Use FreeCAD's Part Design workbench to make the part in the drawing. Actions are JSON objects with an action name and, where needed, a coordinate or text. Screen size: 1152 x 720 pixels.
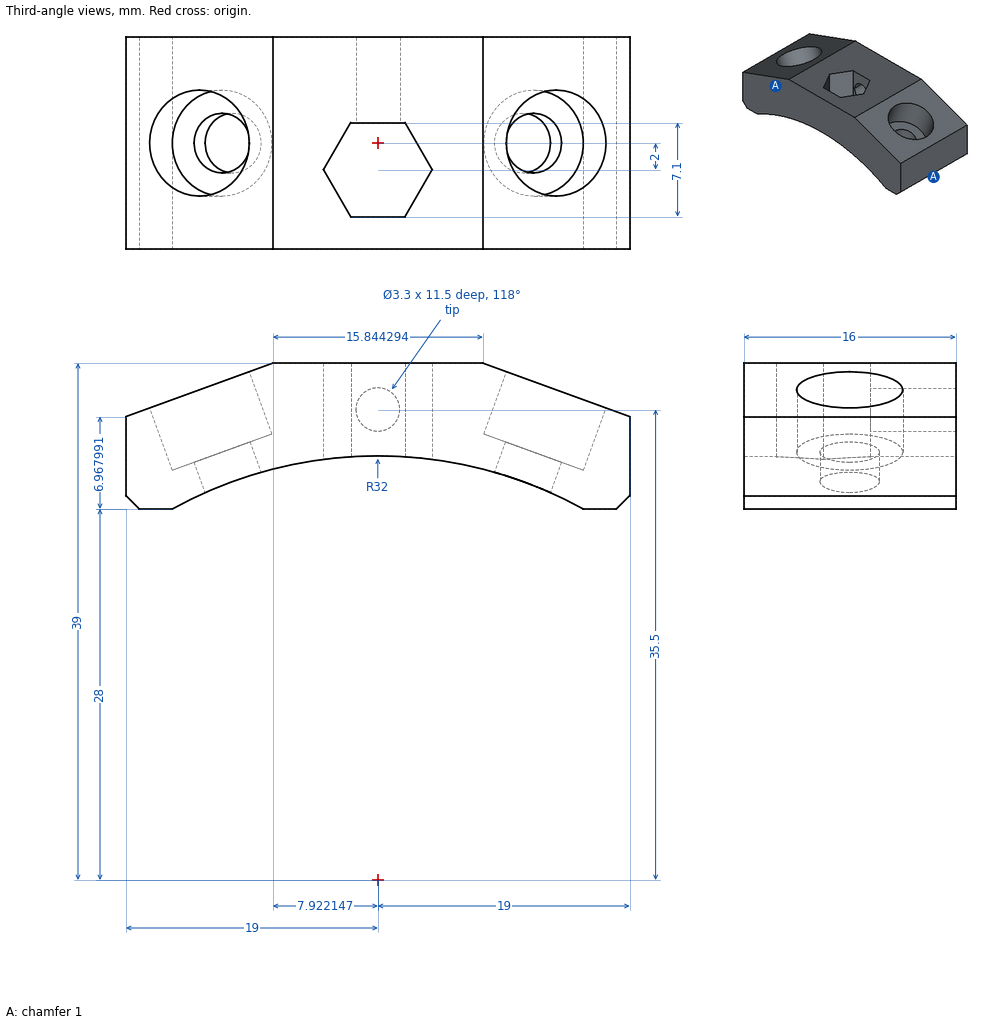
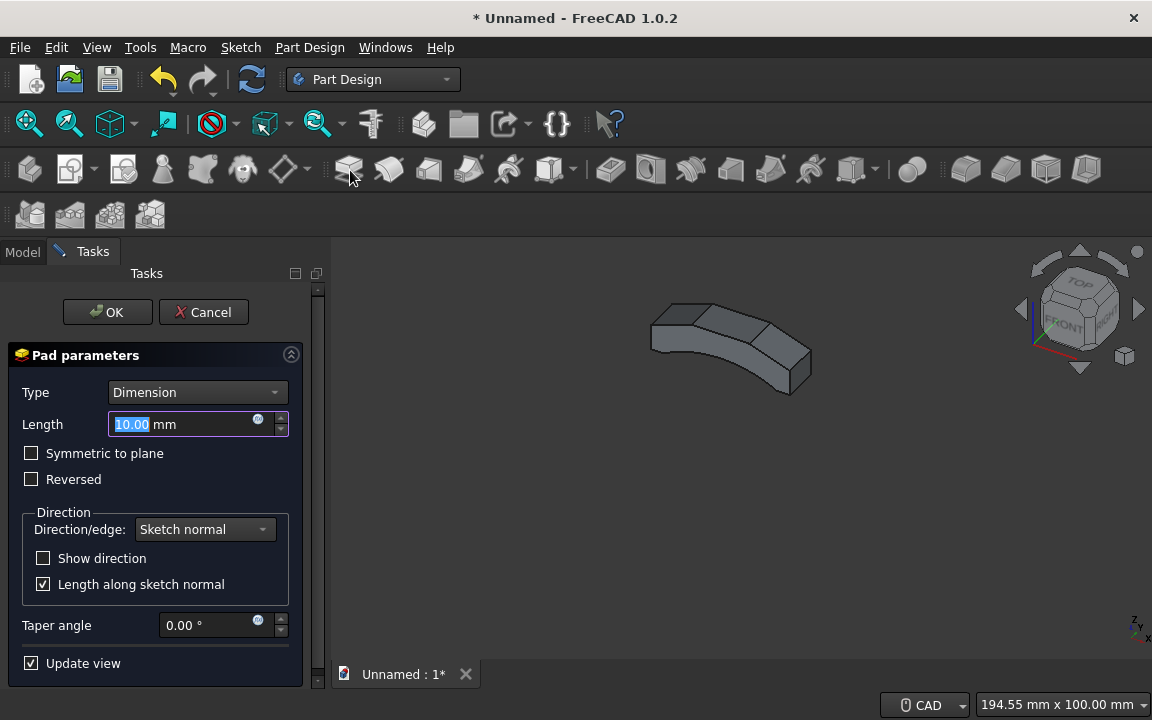
{"action": "type", "text": "16"}
{"action": "key", "text": "Tab"}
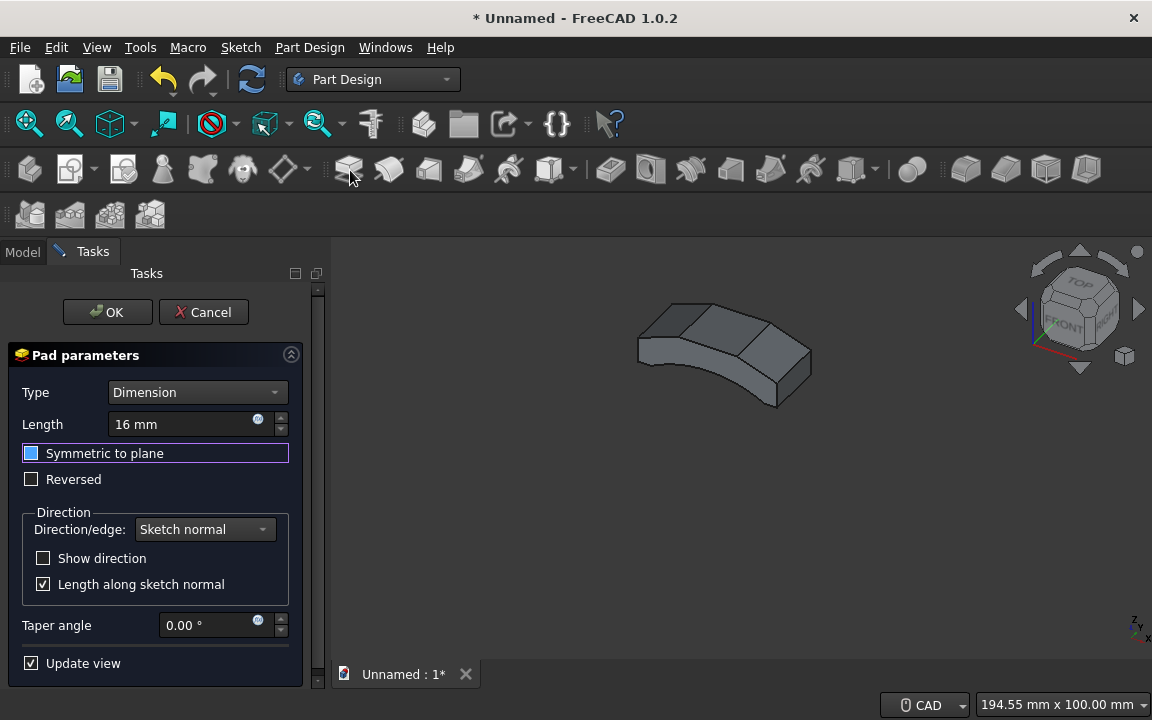
{"action": "left_click", "coordinate": [30, 453]}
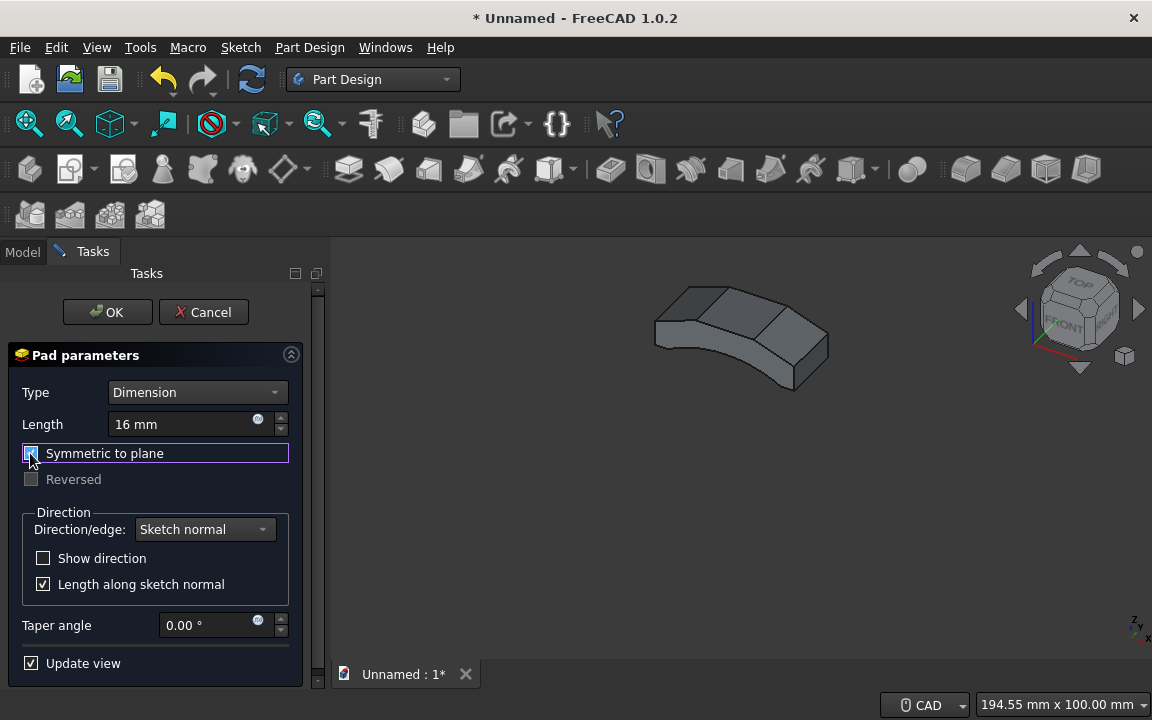
{"action": "left_click", "coordinate": [108, 312]}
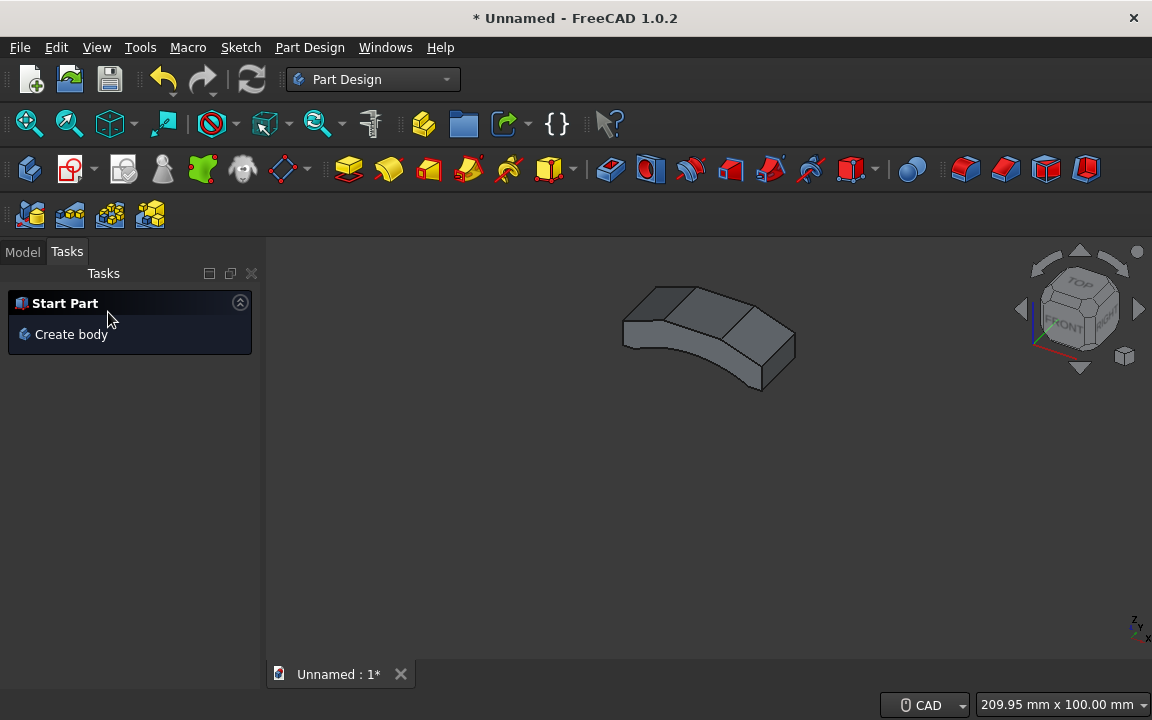
{"action": "left_click", "coordinate": [30, 124]}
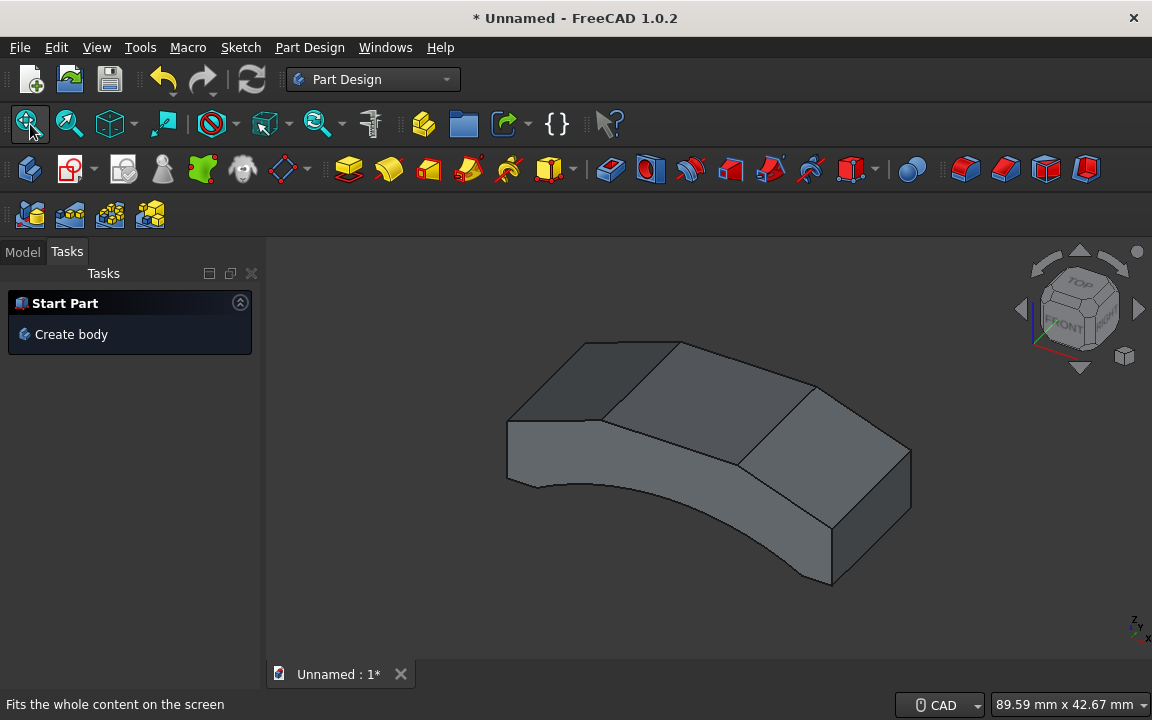
{"action": "left_click", "coordinate": [709, 402]}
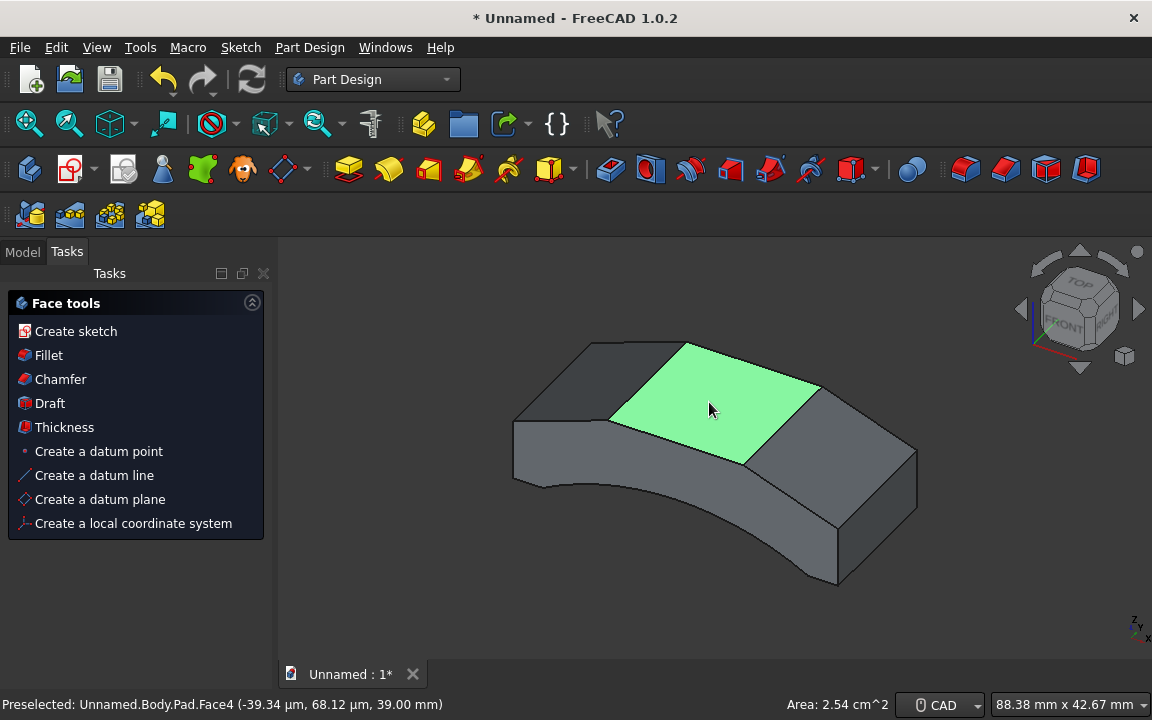
{"action": "left_click", "coordinate": [70, 170]}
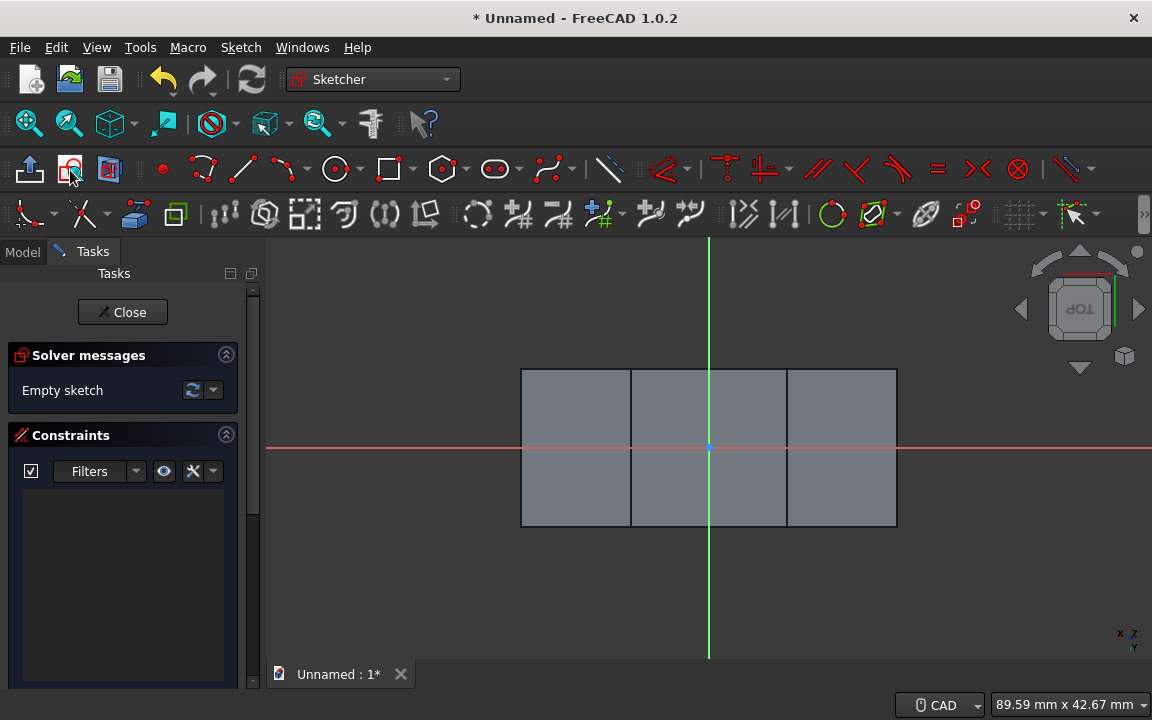
{"action": "scroll", "coordinate": [731, 422], "scroll_direction": "up", "scroll_amount": 7}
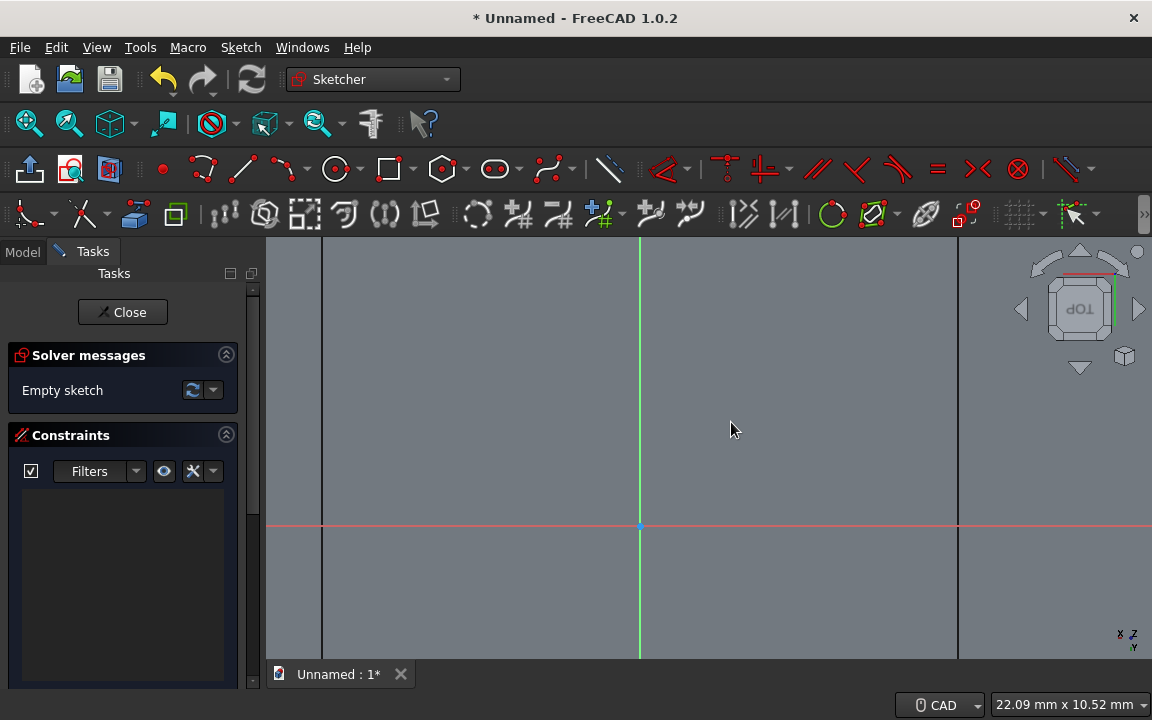
{"action": "key", "text": "g p 6"}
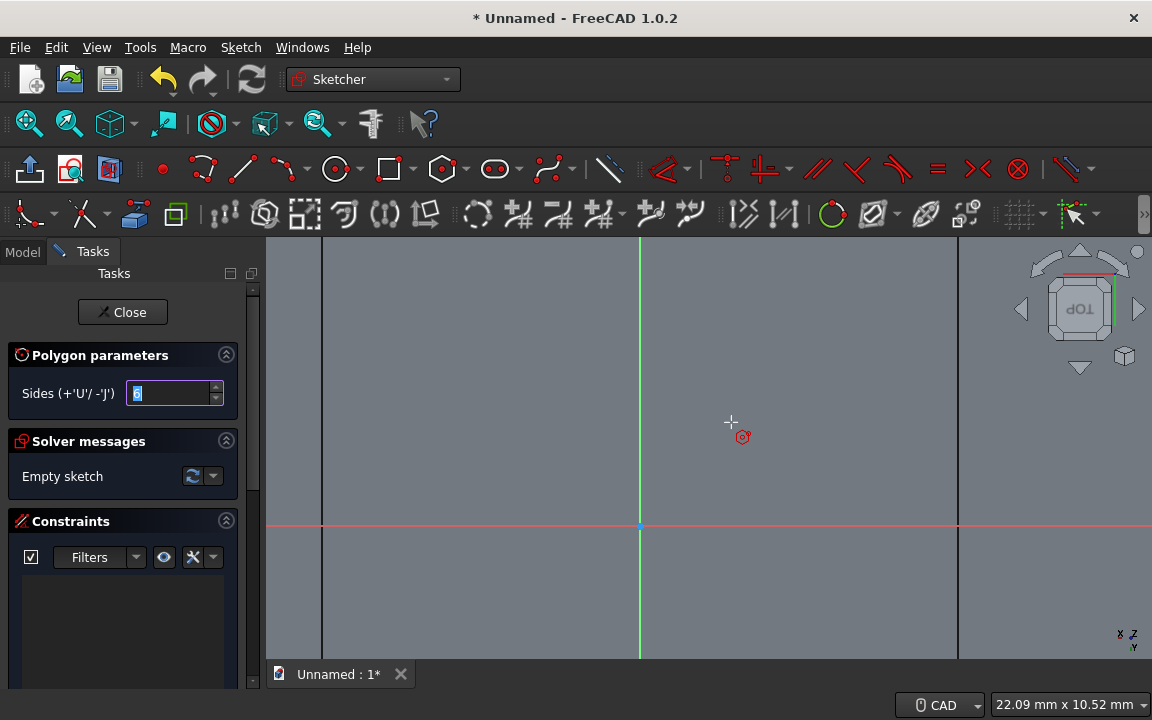
{"action": "left_click", "coordinate": [640, 446]}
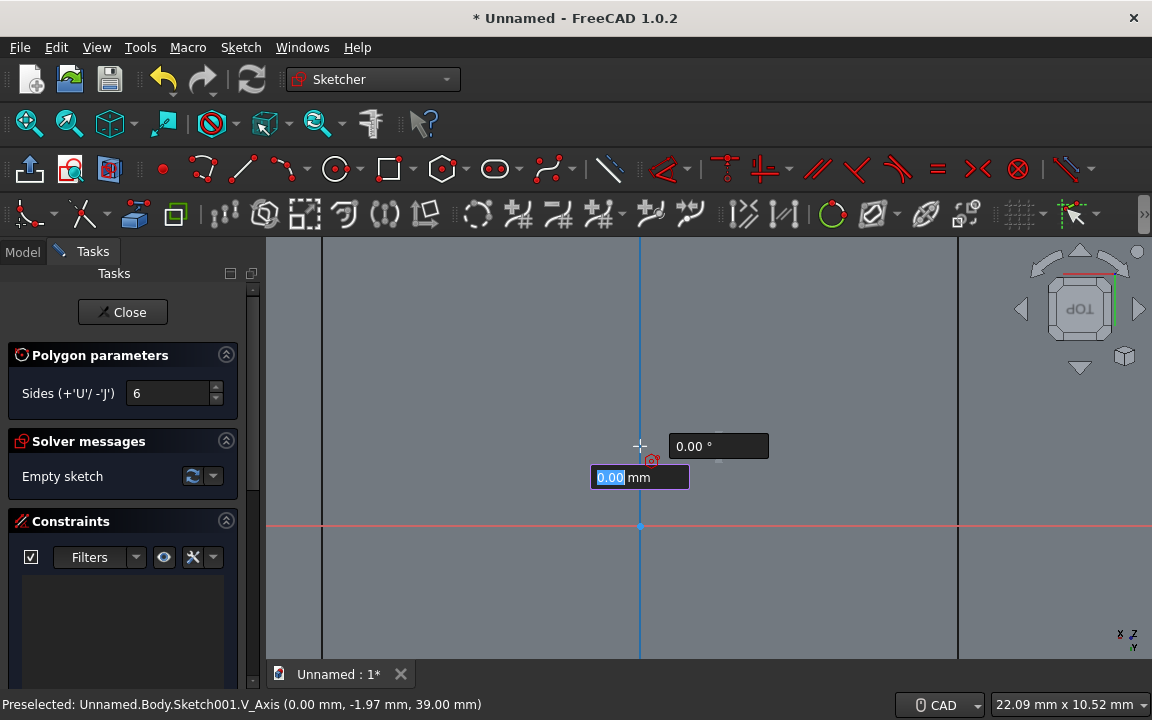
{"action": "left_click", "coordinate": [476, 446]}
{"action": "right_click", "coordinate": [476, 446]}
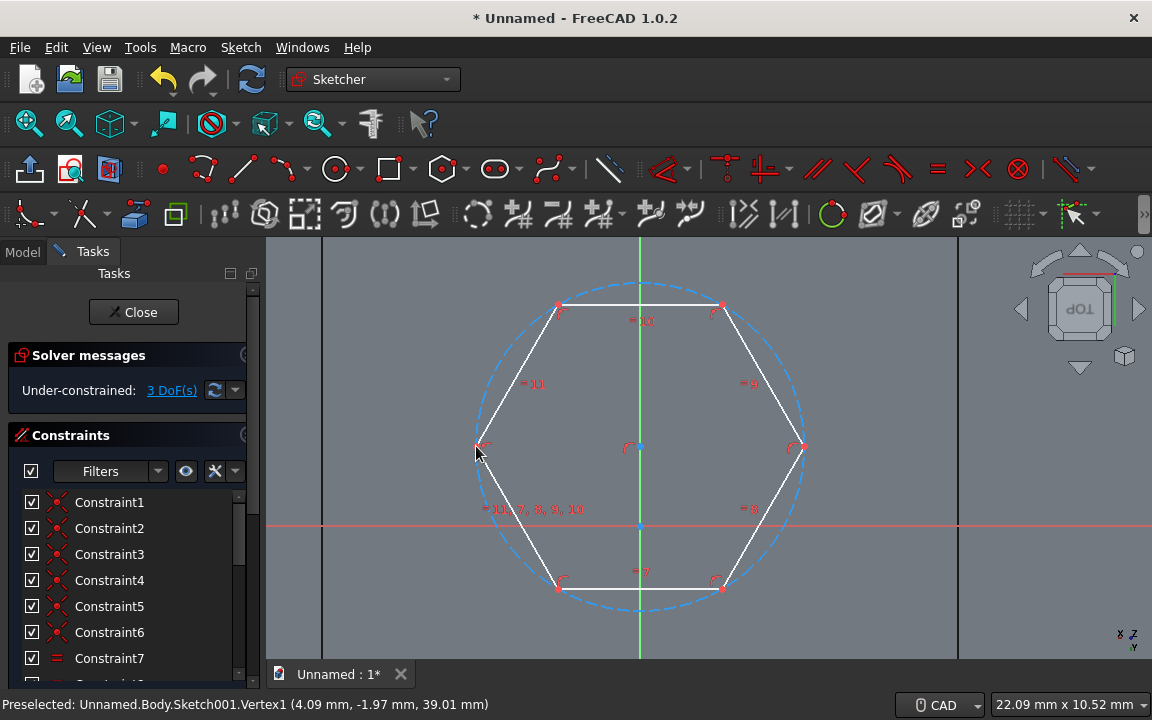
{"action": "left_click", "coordinate": [607, 589]}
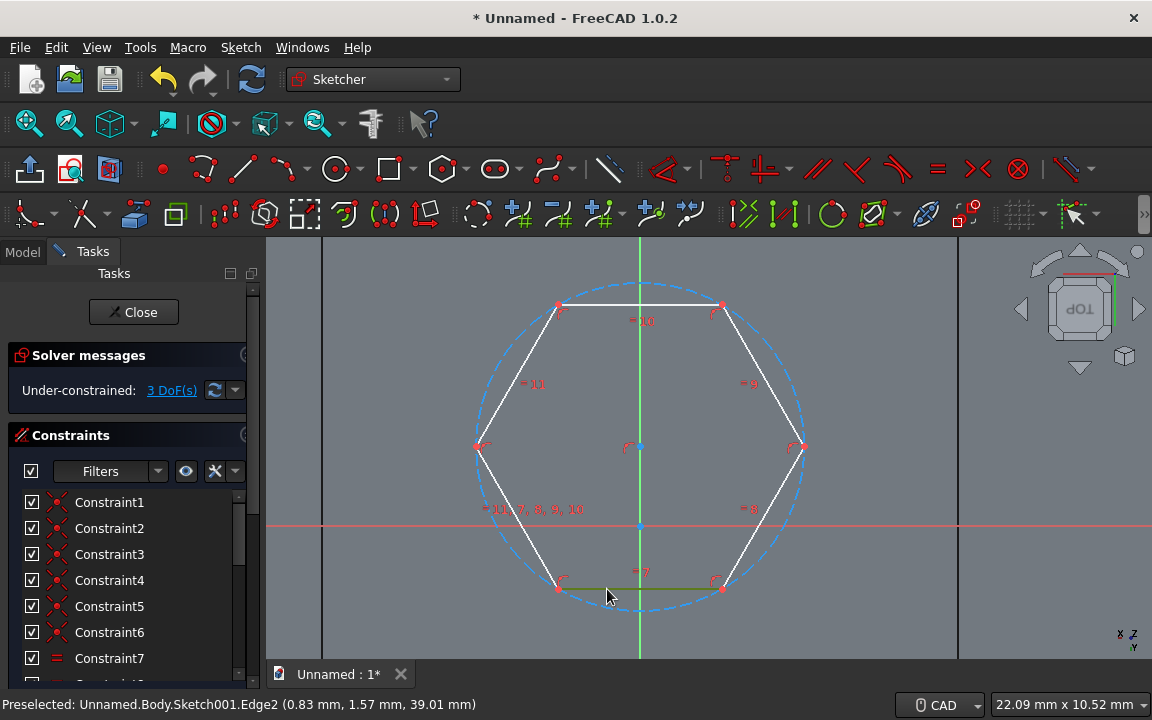
{"action": "key", "text": "h"}